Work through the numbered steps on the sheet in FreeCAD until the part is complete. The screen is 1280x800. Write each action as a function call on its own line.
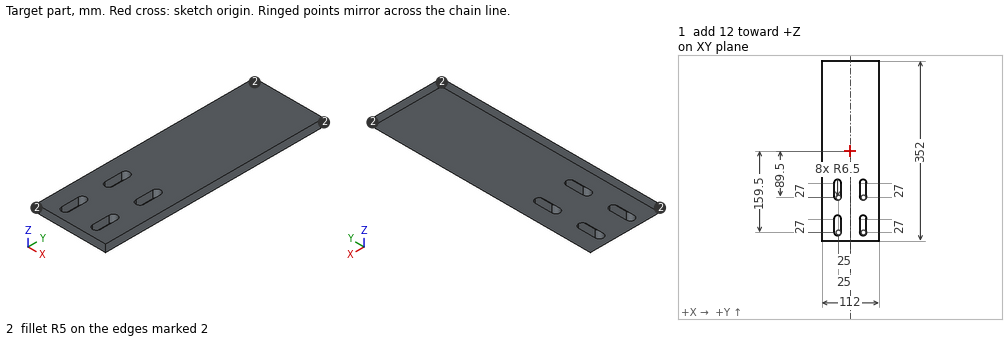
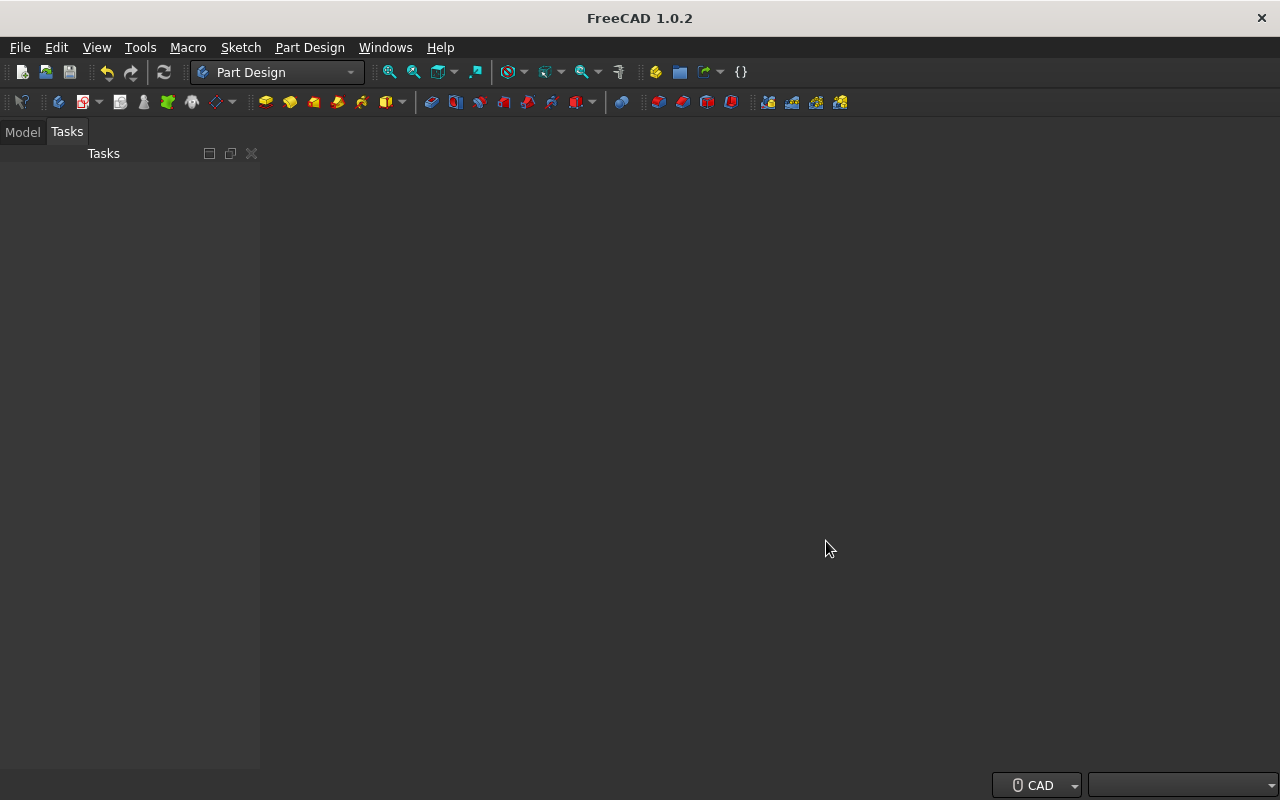
click(22, 72)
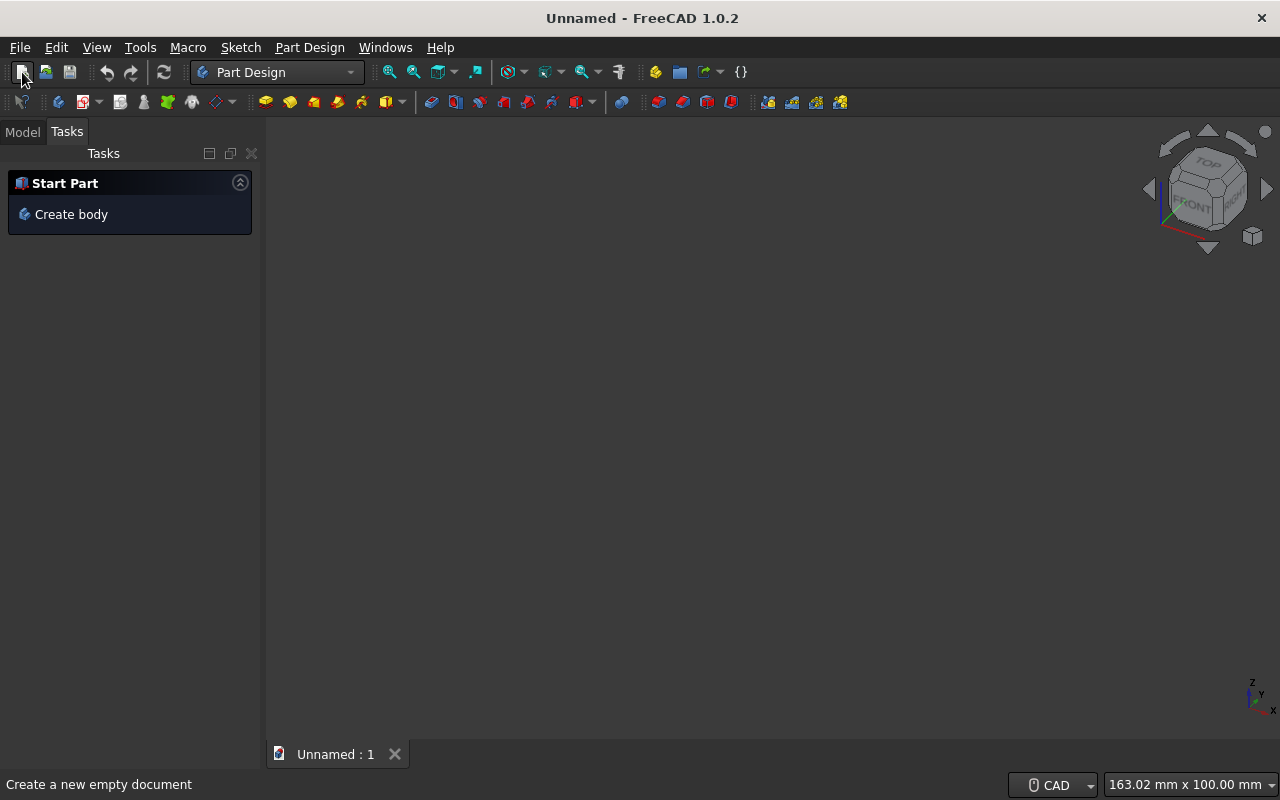
click(84, 102)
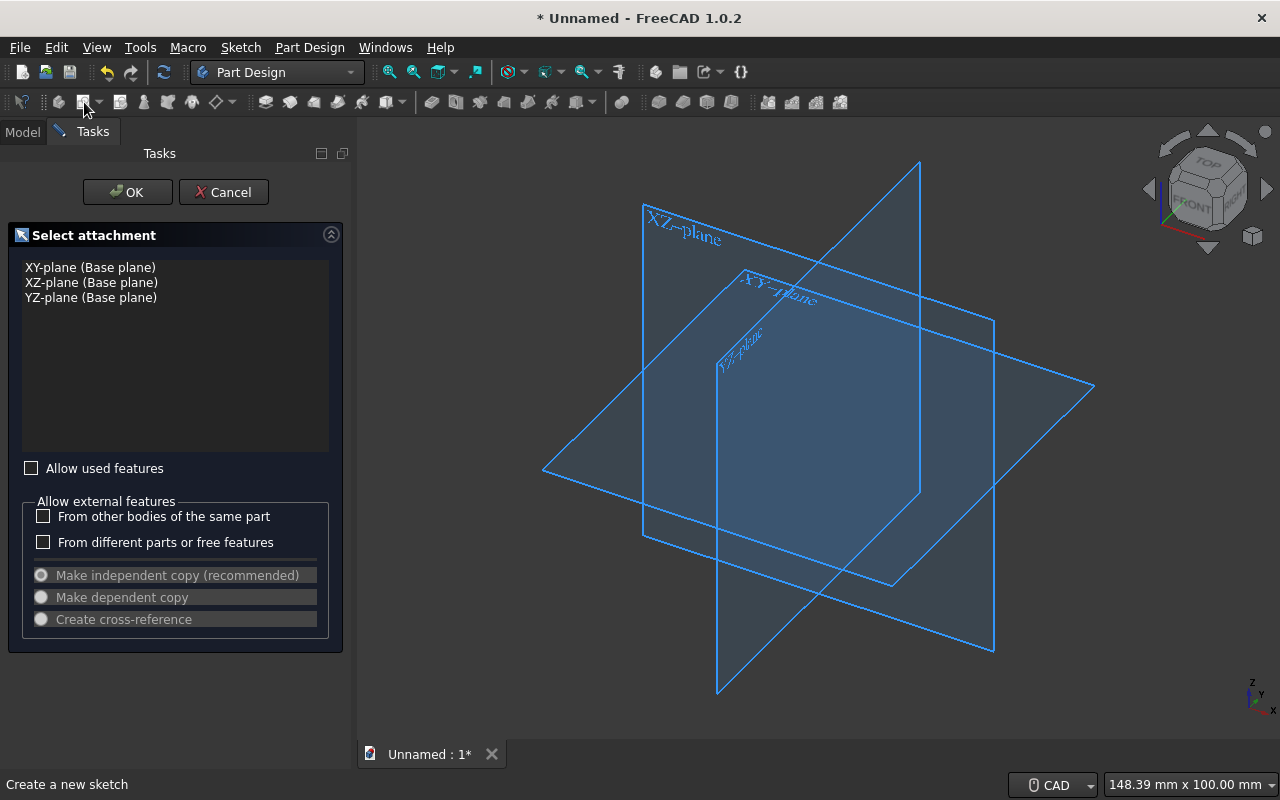
click(82, 268)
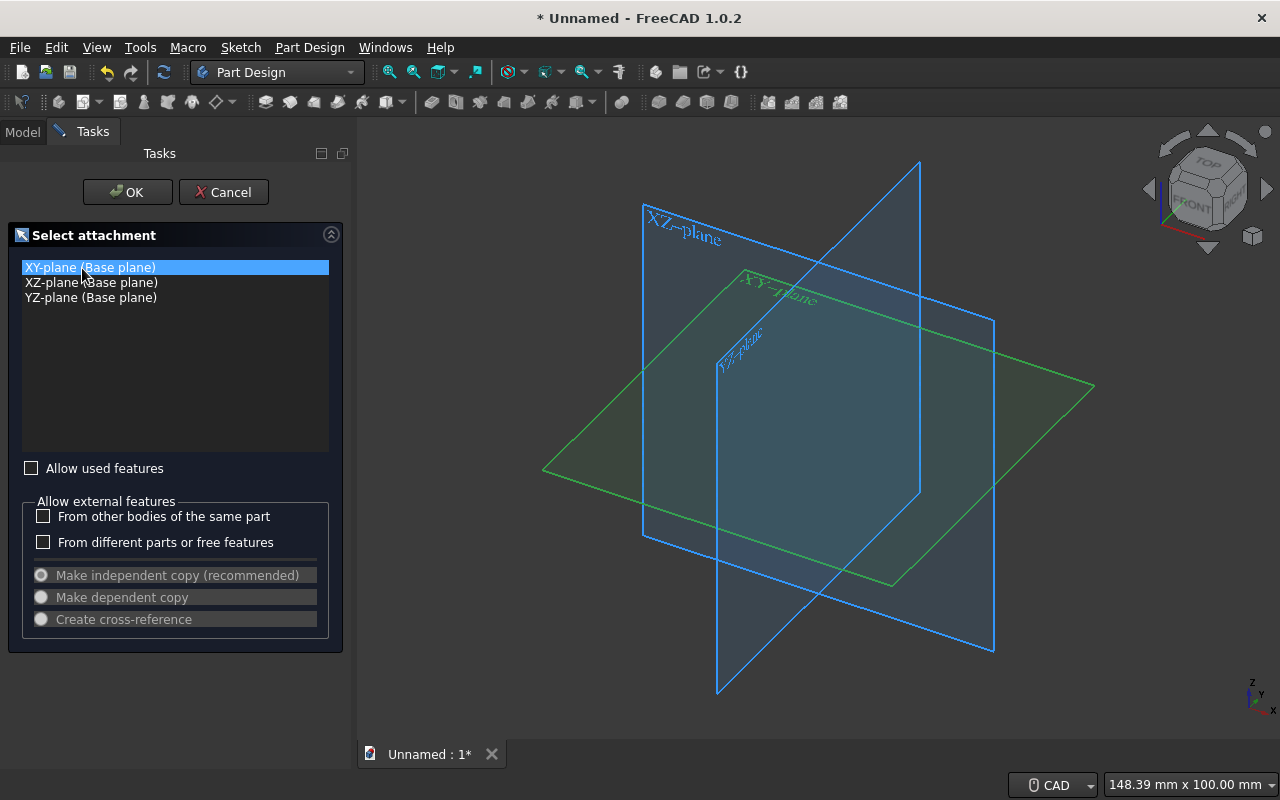
click(128, 192)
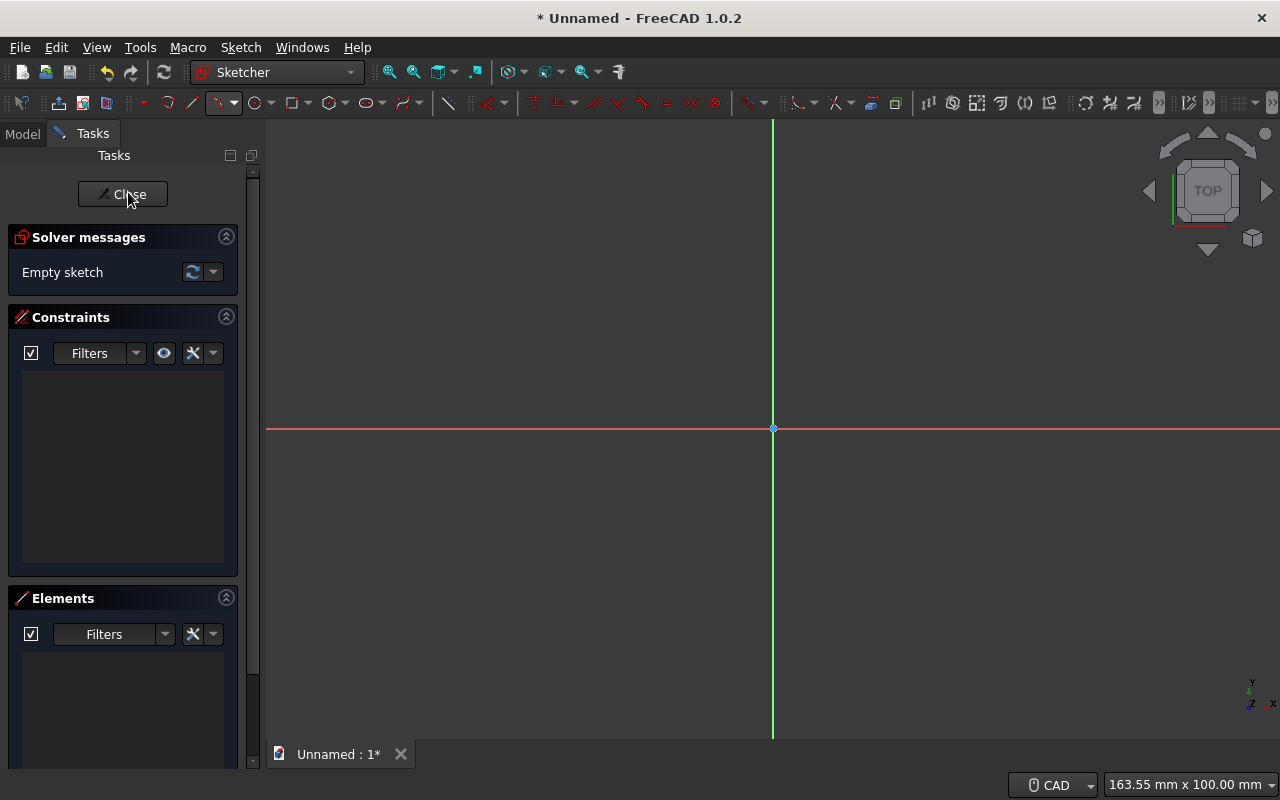
scroll(691, 429, down, 9)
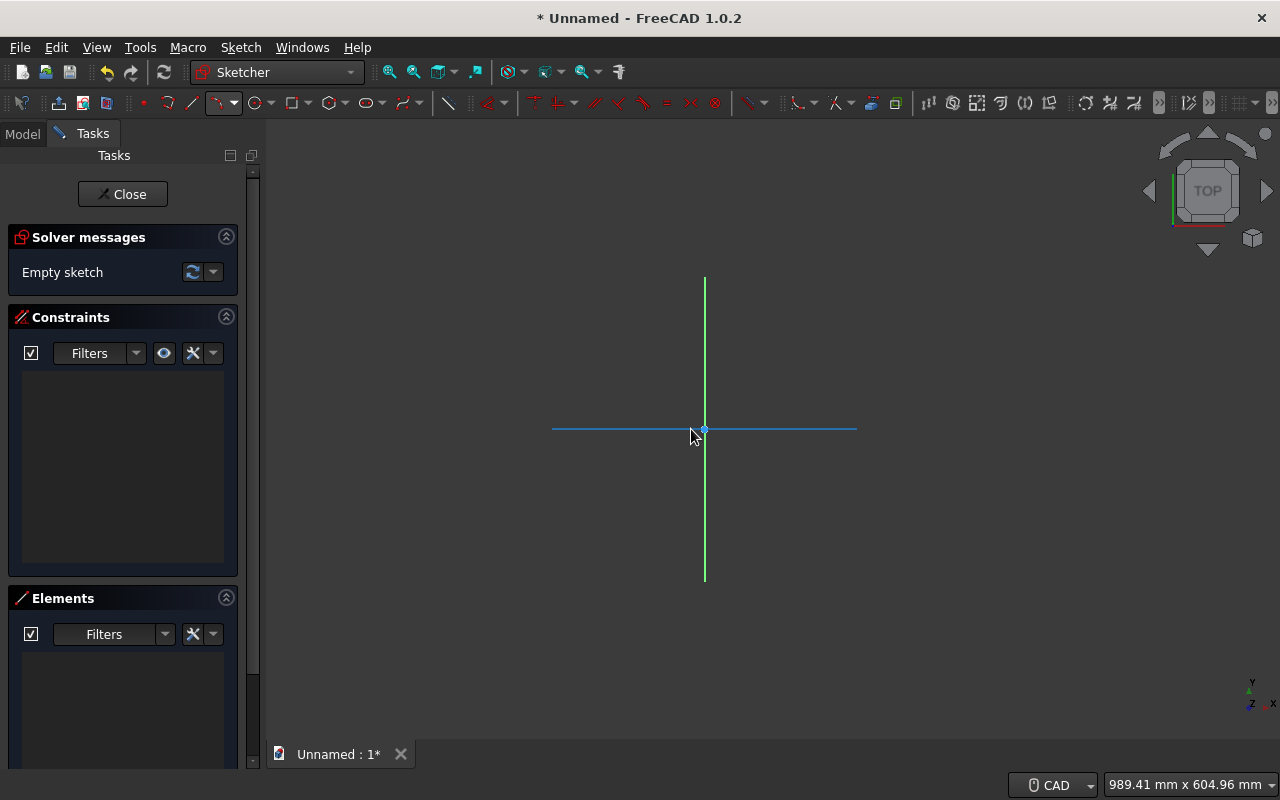
click(310, 104)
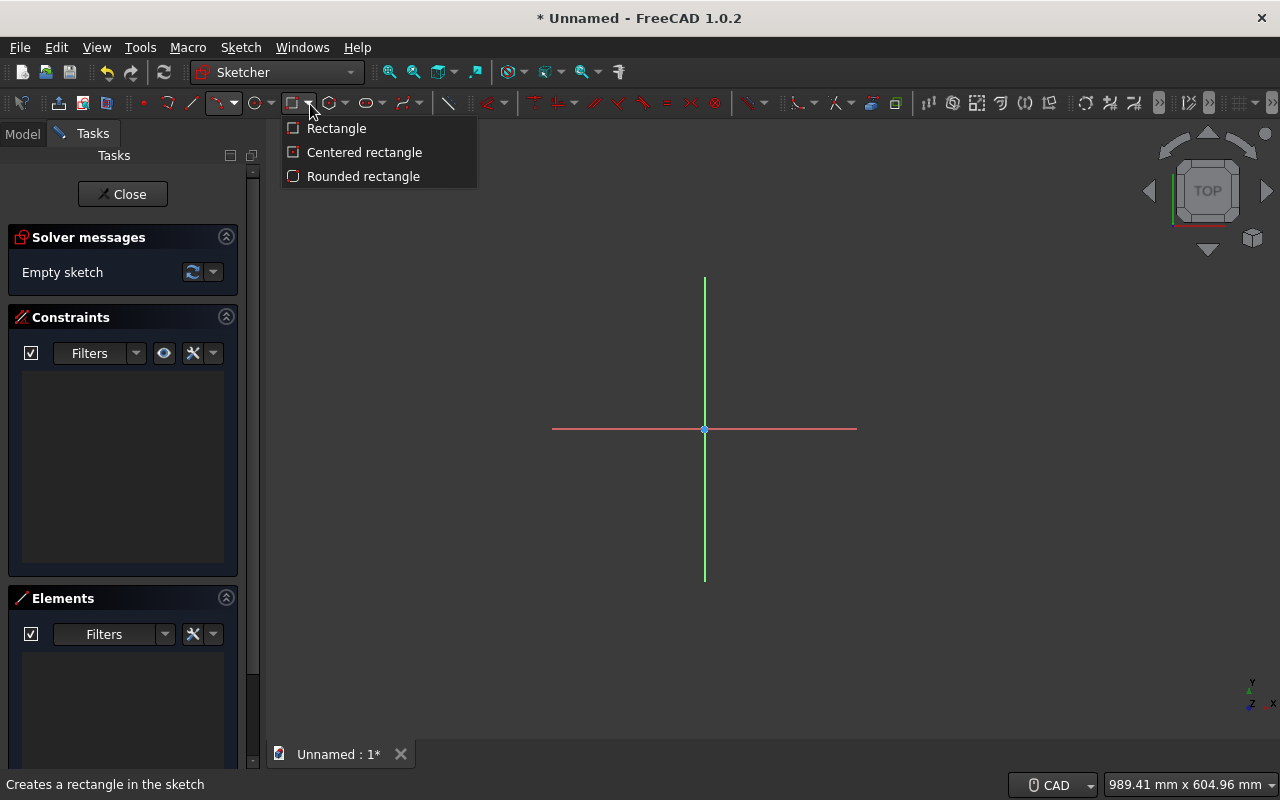
click(380, 152)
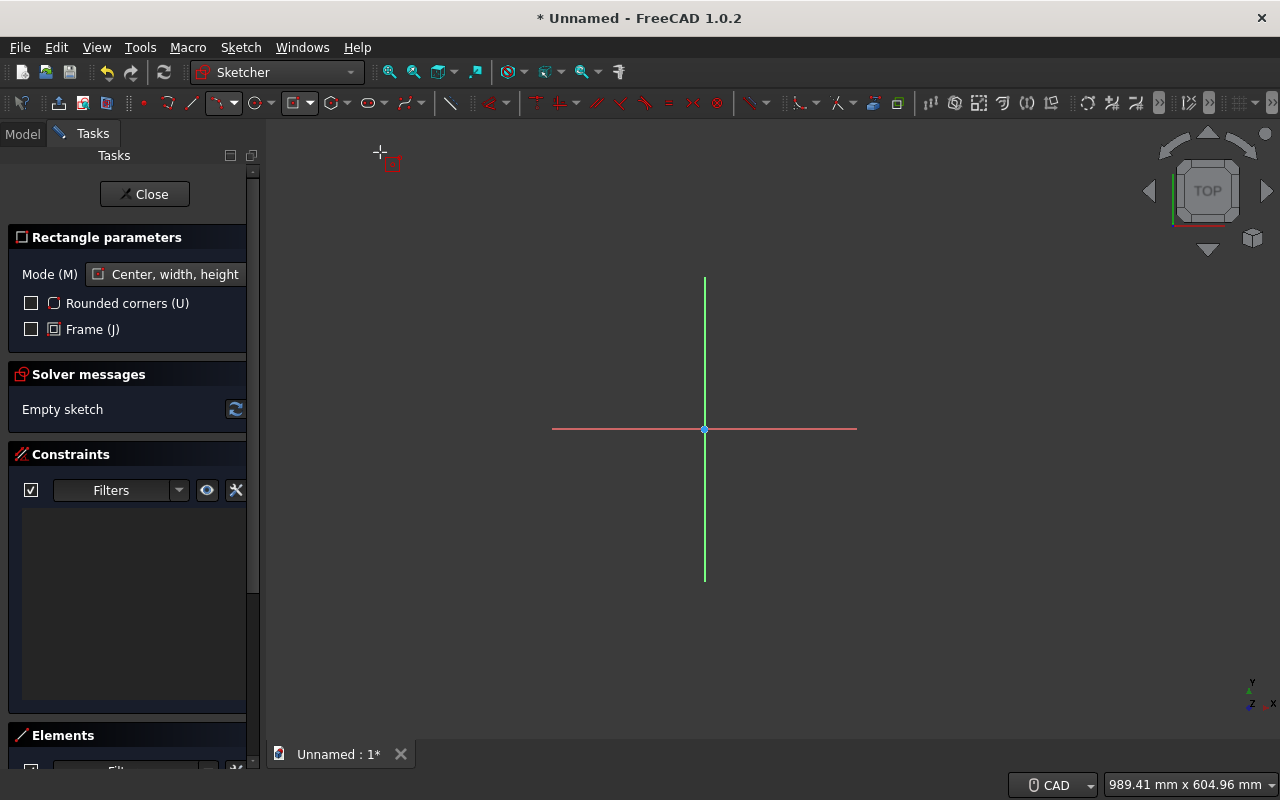
click(705, 429)
click(762, 249)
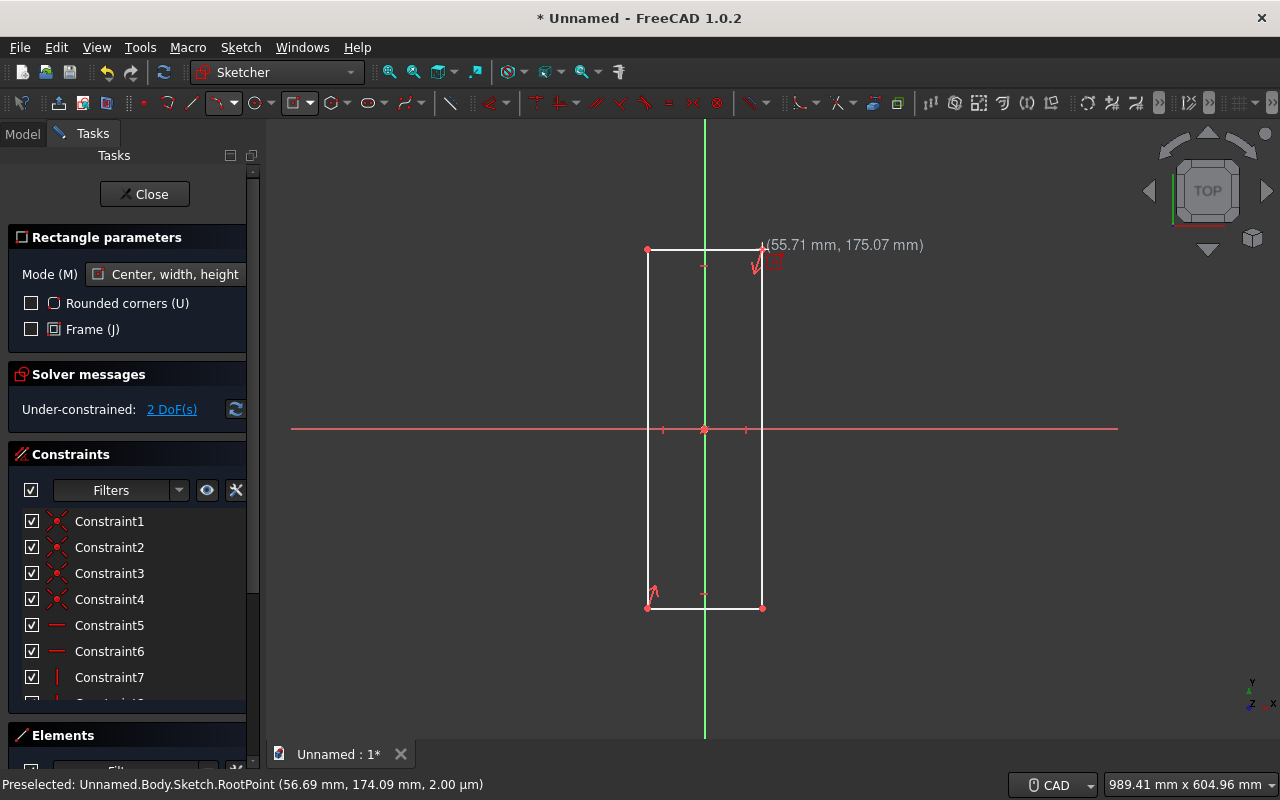
click(368, 104)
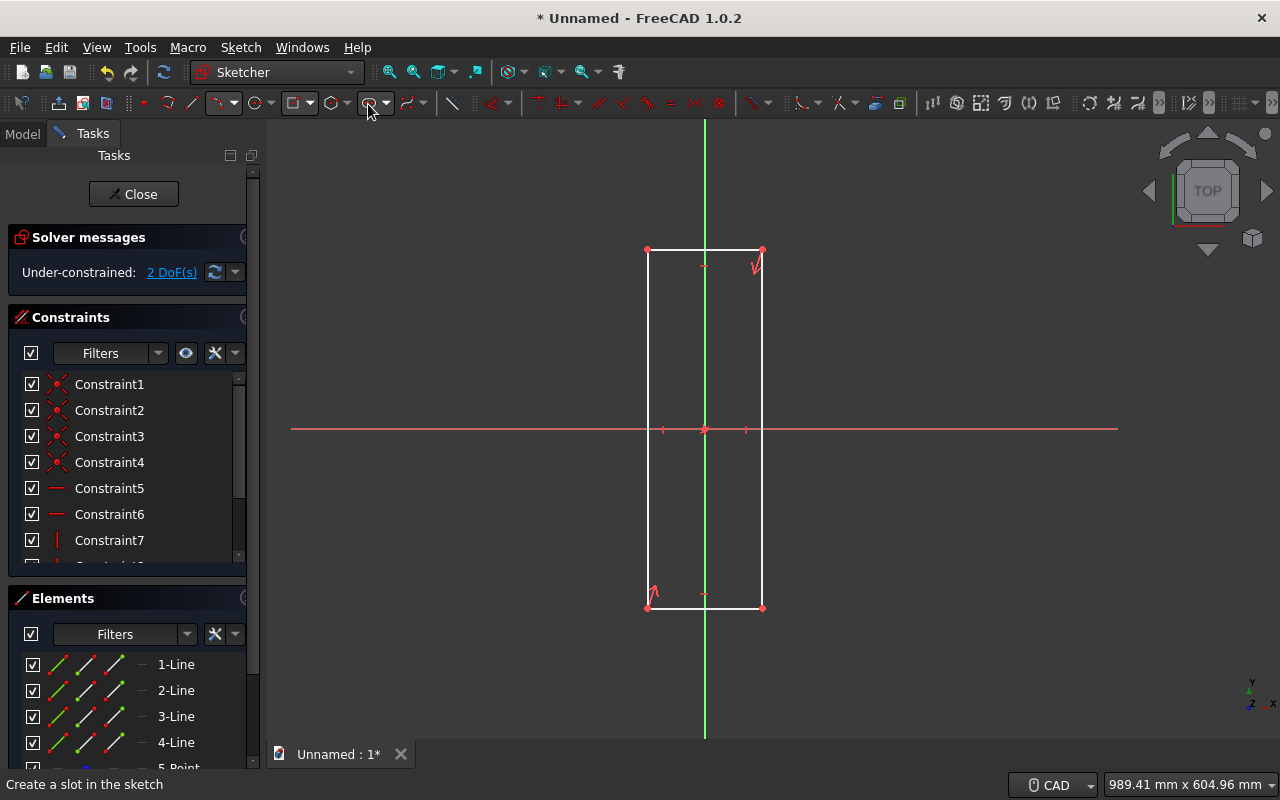
scroll(679, 593, up, 7)